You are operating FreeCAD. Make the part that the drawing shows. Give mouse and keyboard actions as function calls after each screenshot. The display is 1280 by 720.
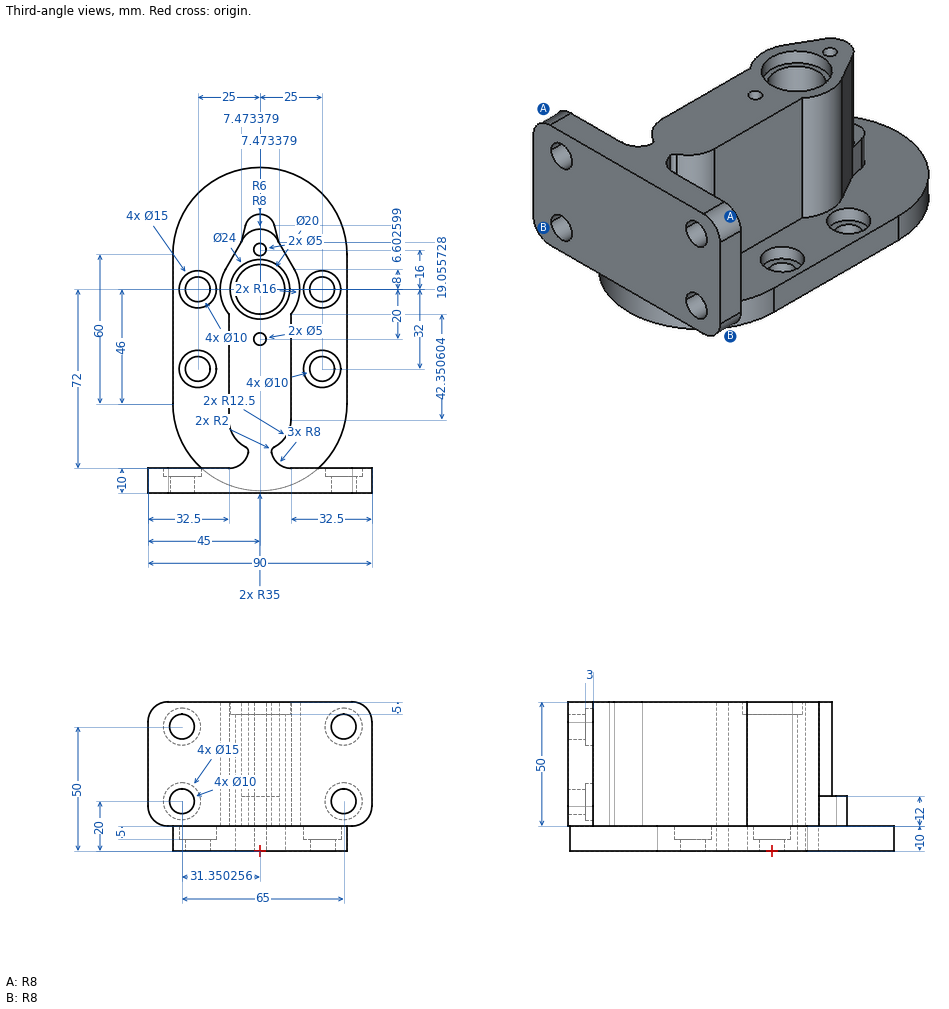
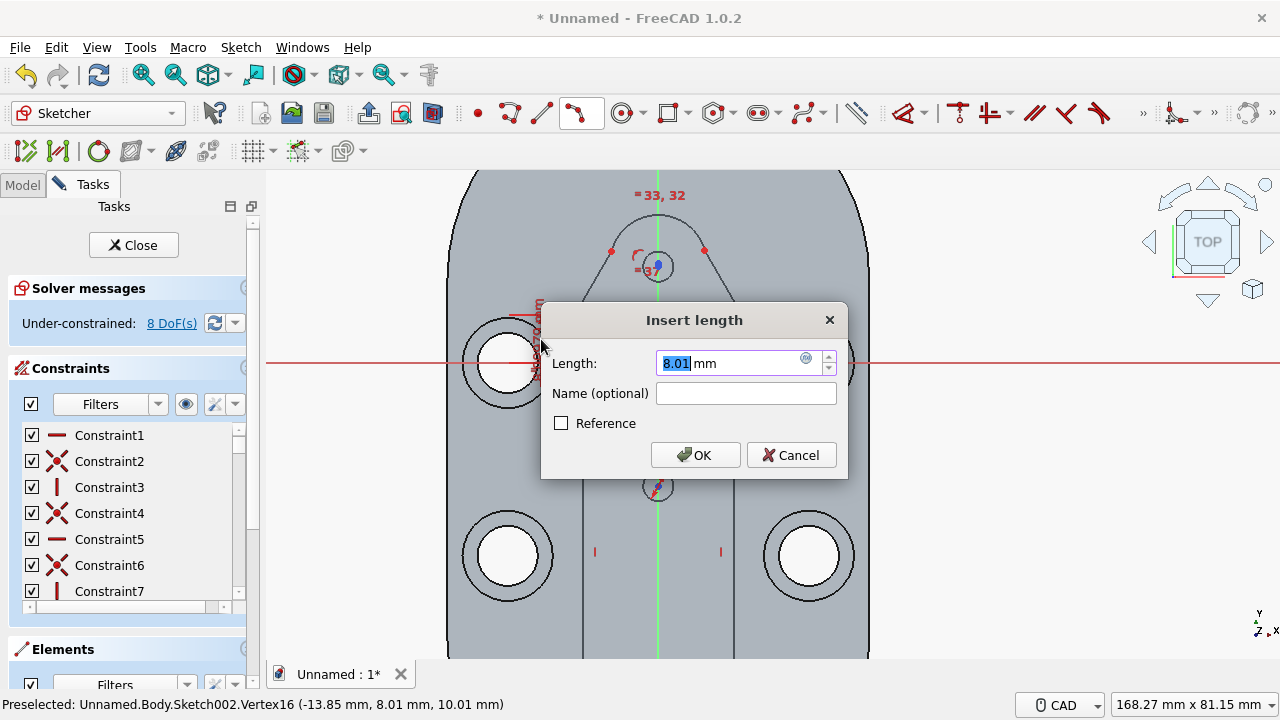
text(8)
key(Return)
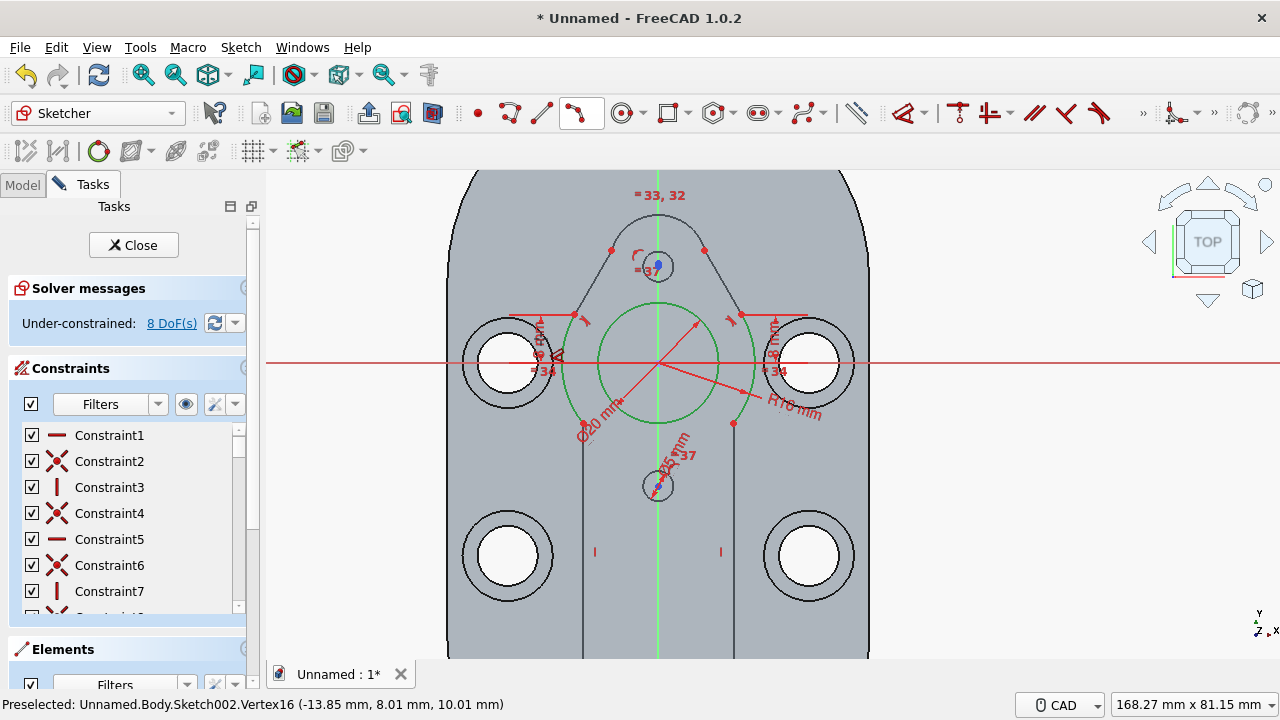
click(658, 486)
click(692, 381)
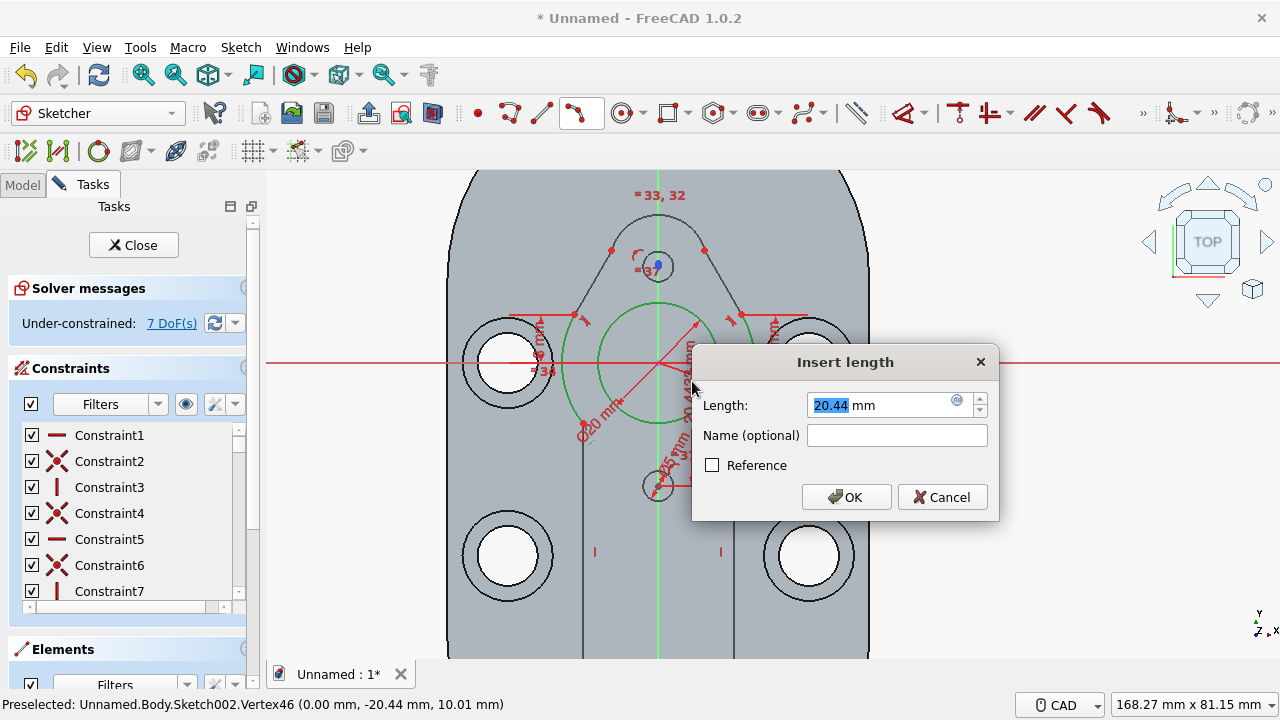
text(20)
key(Return)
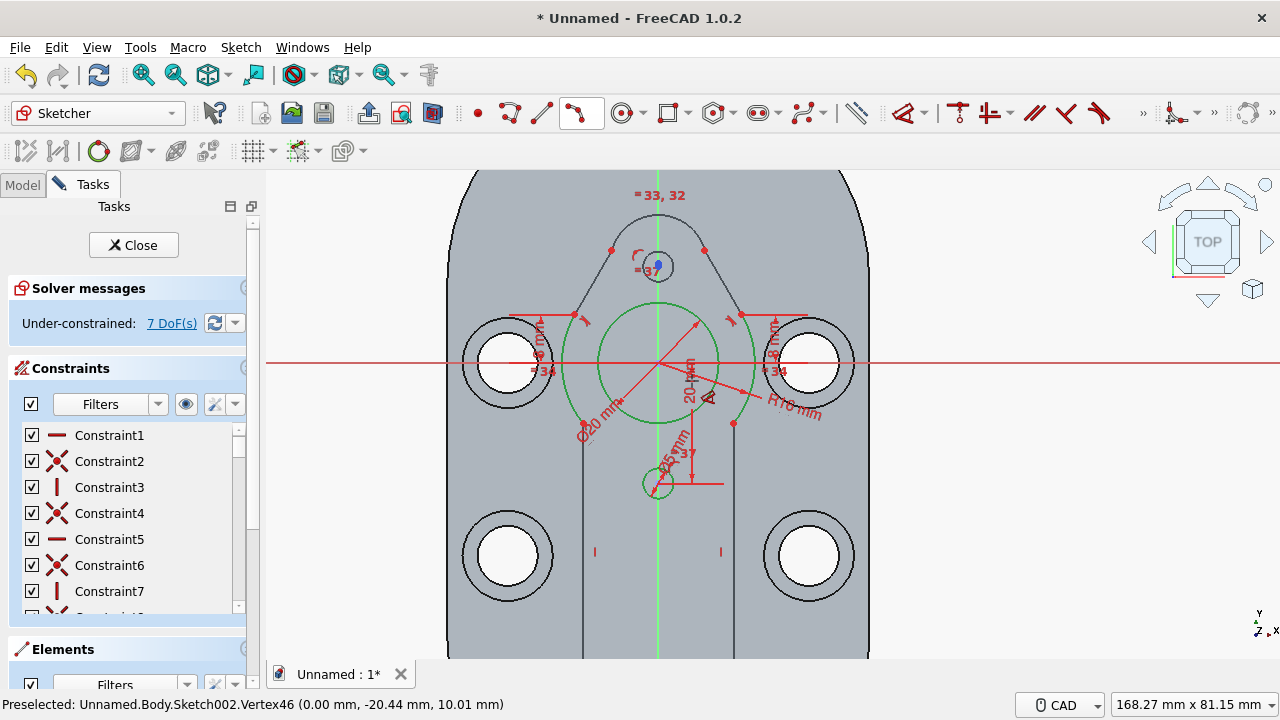
scroll(658, 267, up, 7)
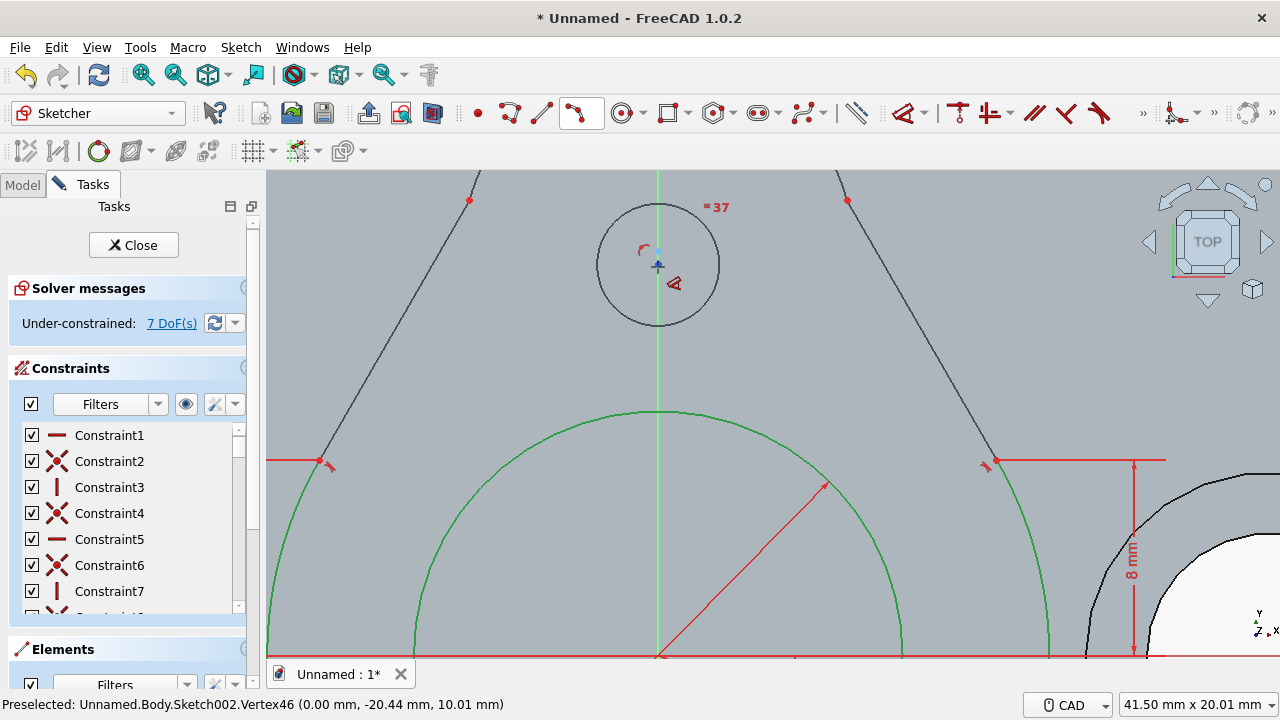
click(658, 265)
click(692, 448)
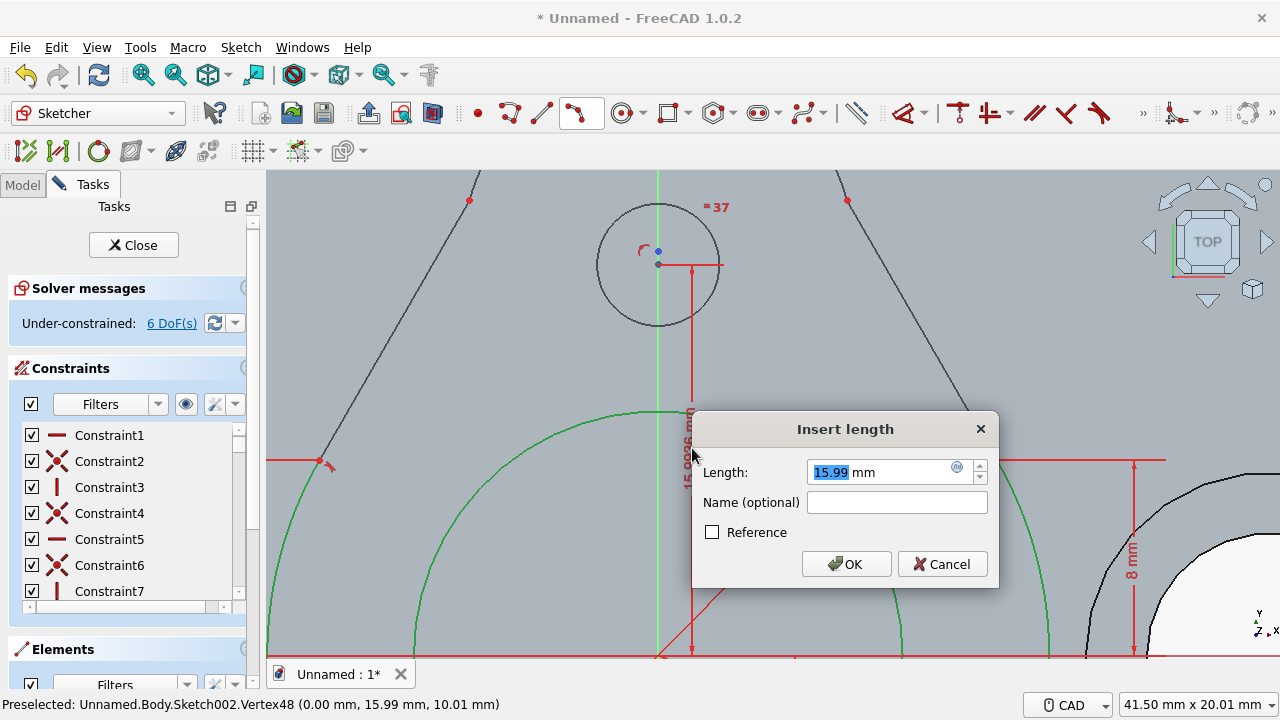
text(16)
key(Return)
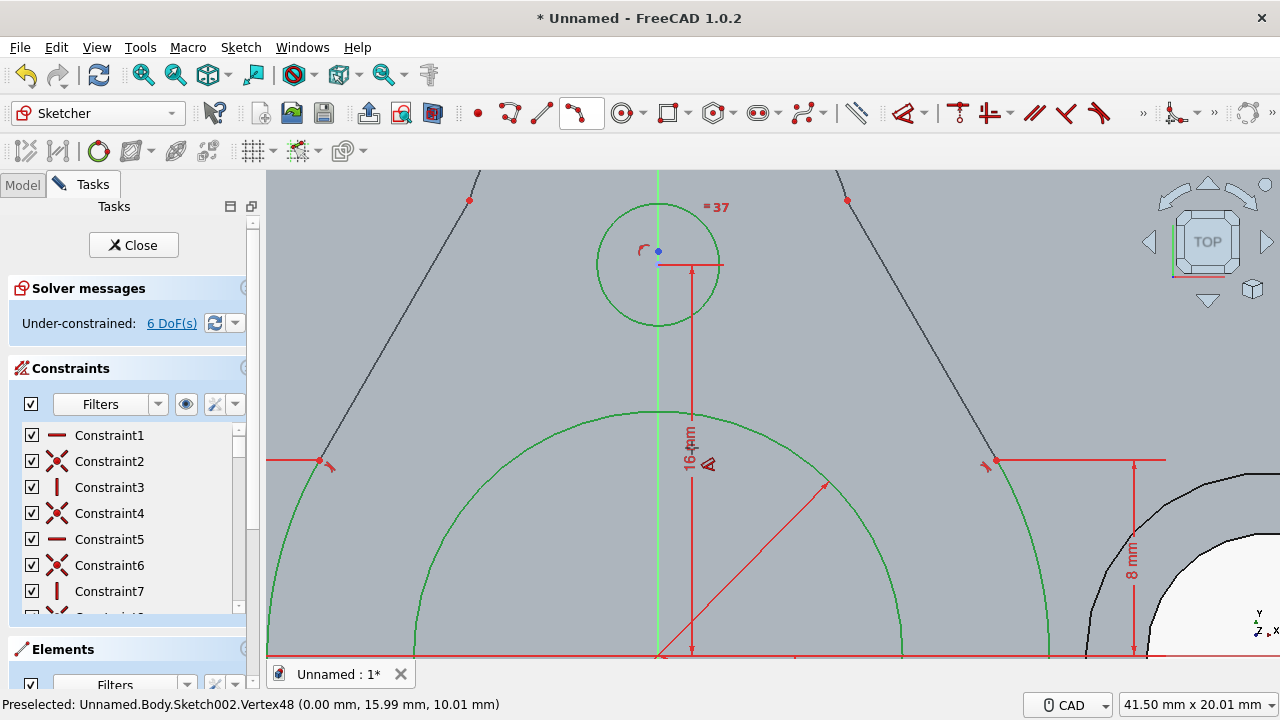
scroll(710, 296, down, 11)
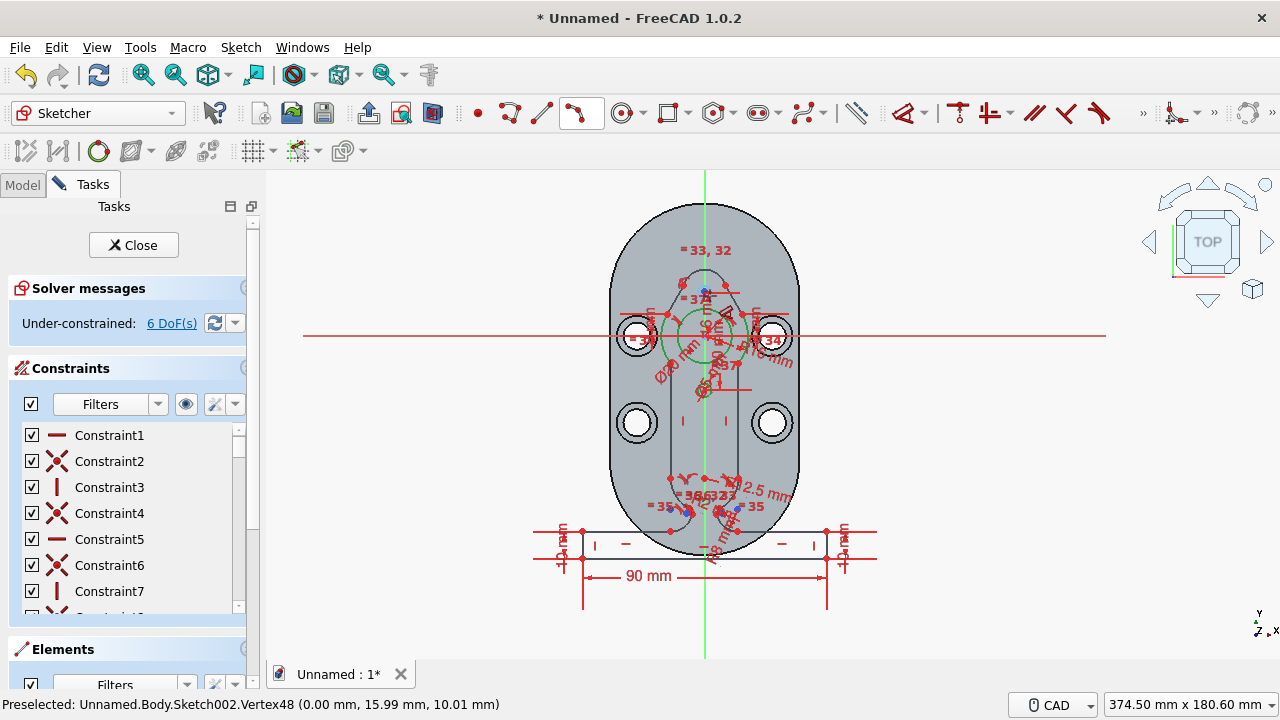
click(671, 532)
click(637, 434)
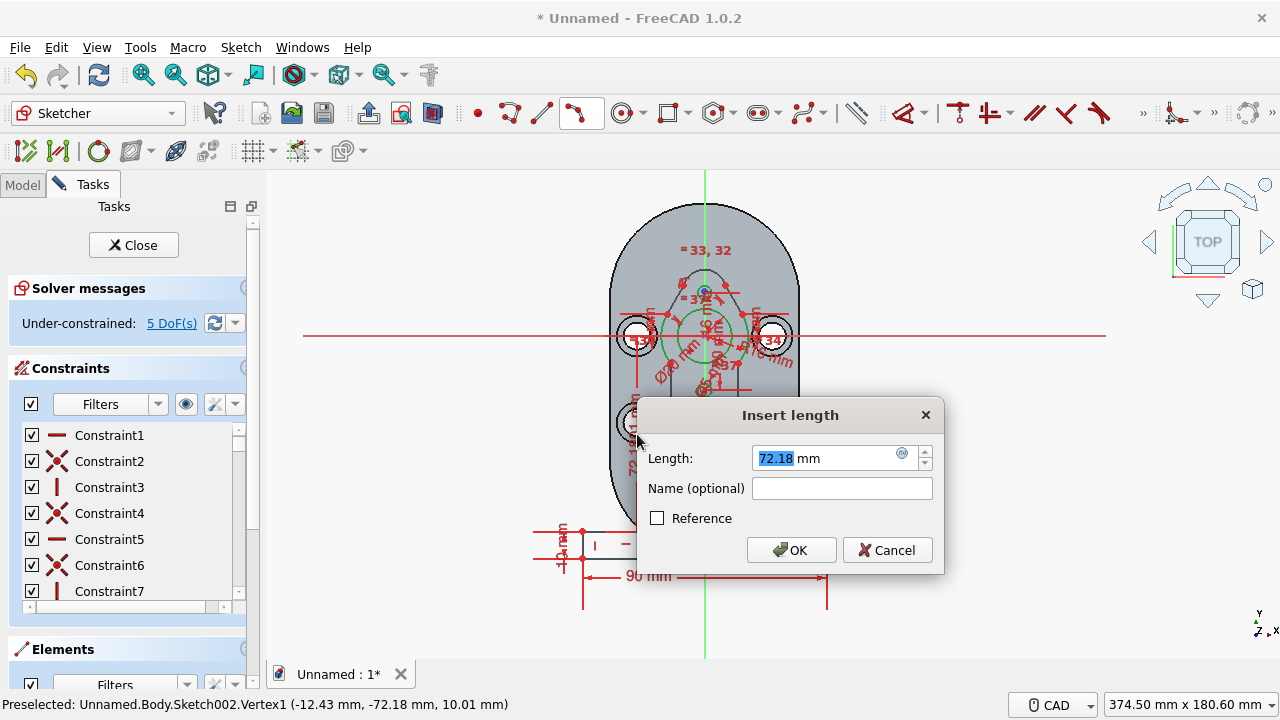
text(72)
key(Return)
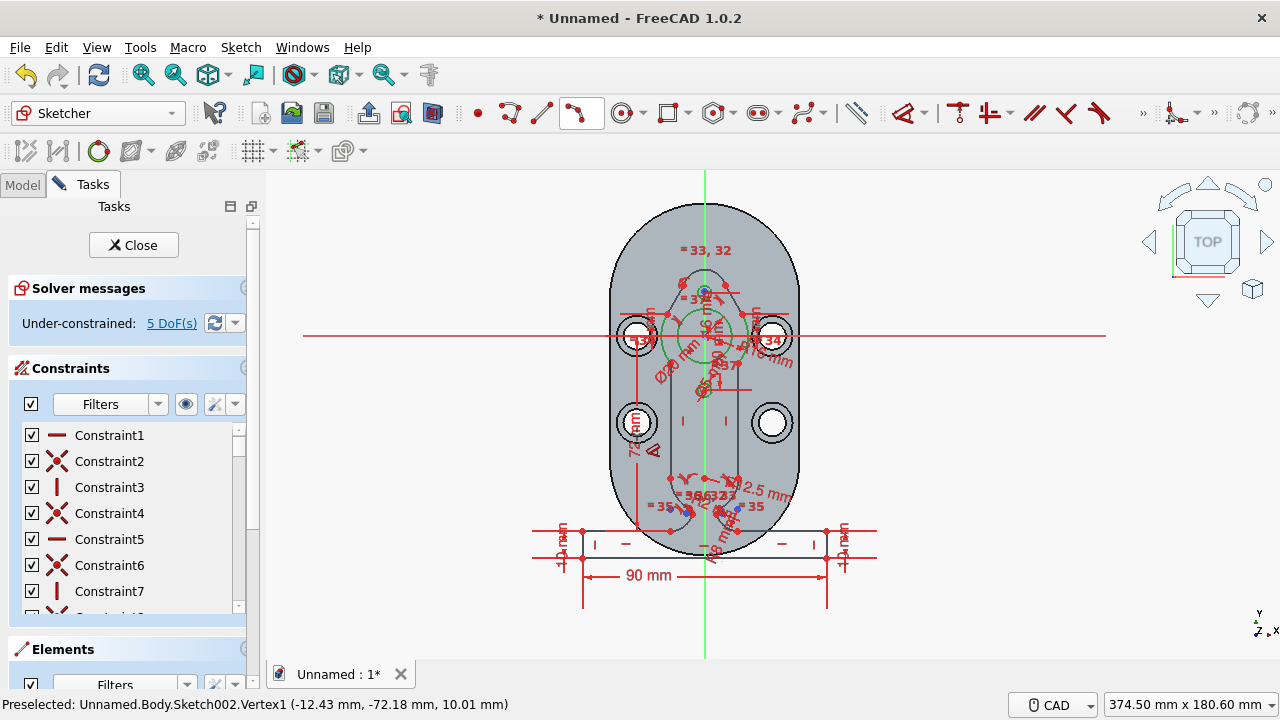
click(583, 531)
click(616, 302)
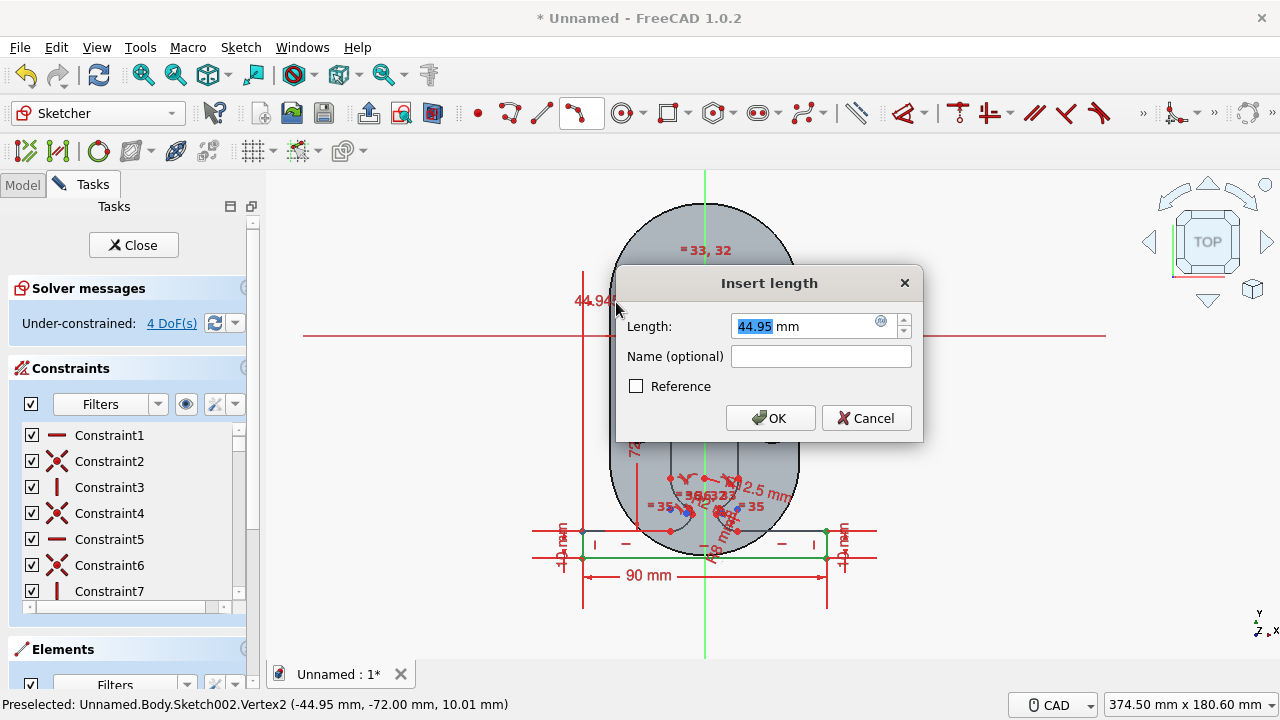
text(45)
key(Return)